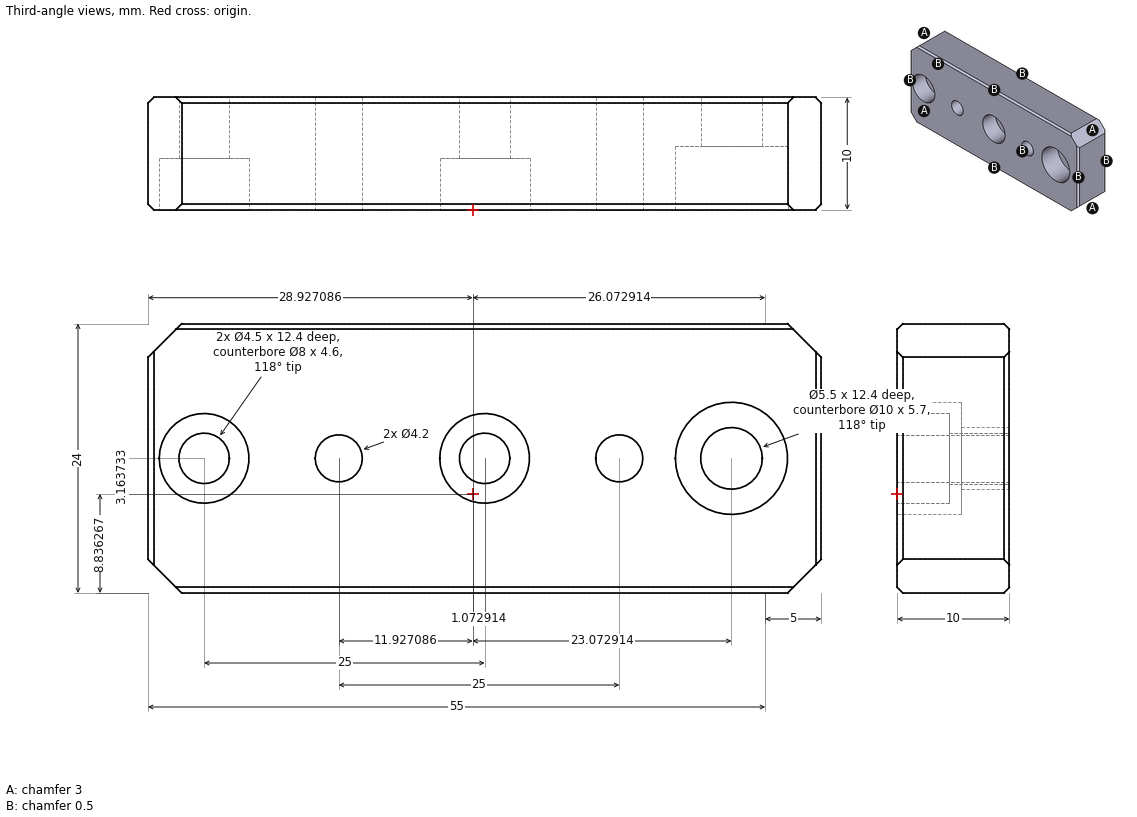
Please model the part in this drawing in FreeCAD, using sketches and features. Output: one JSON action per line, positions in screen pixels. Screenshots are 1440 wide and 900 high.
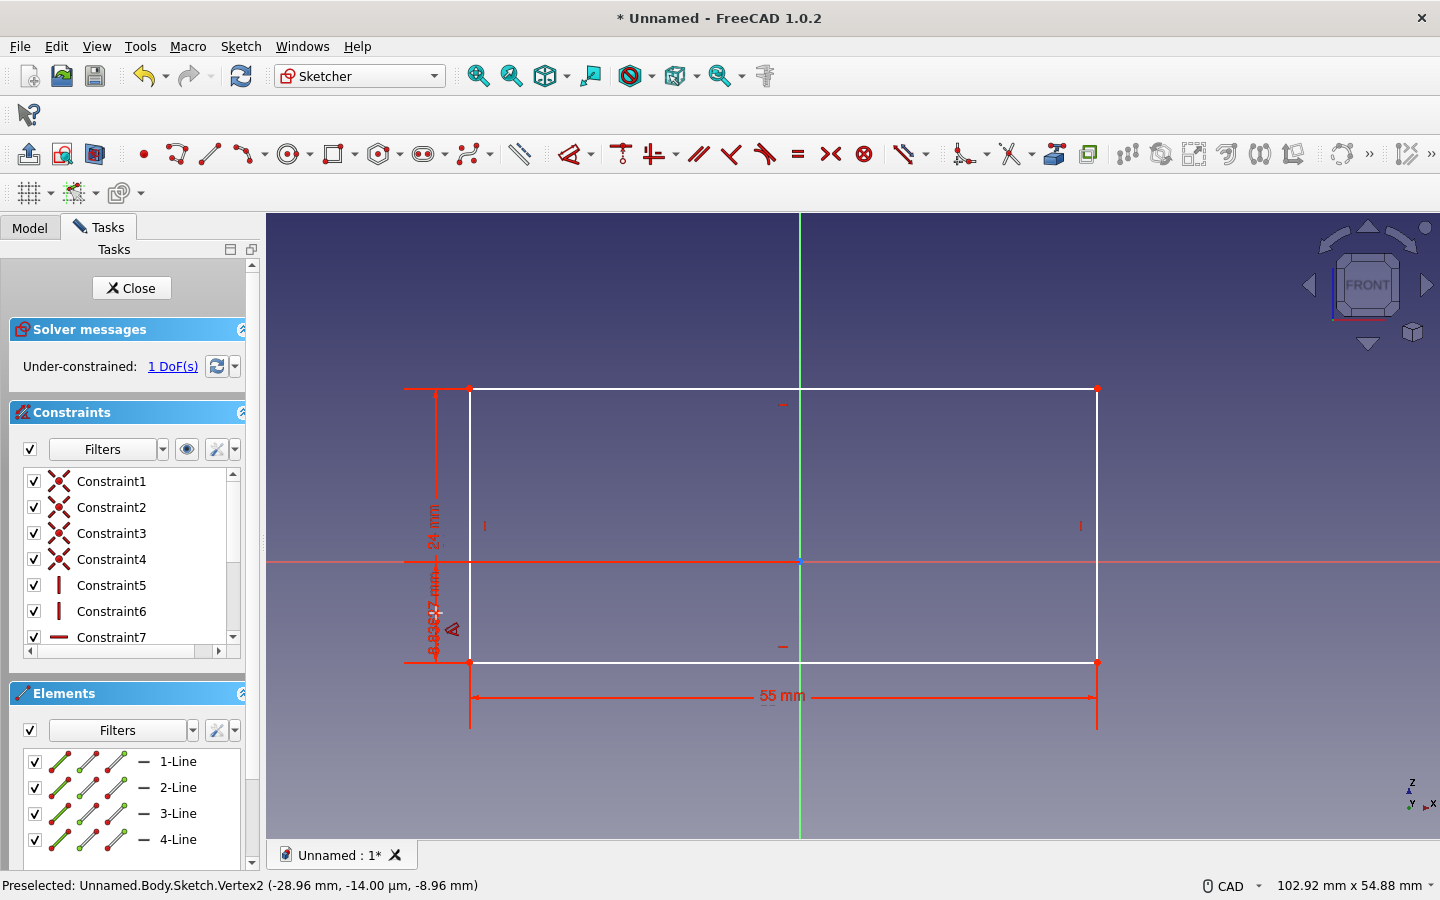
{"action": "left_click", "coordinate": [470, 389]}
{"action": "left_click", "coordinate": [635, 355]}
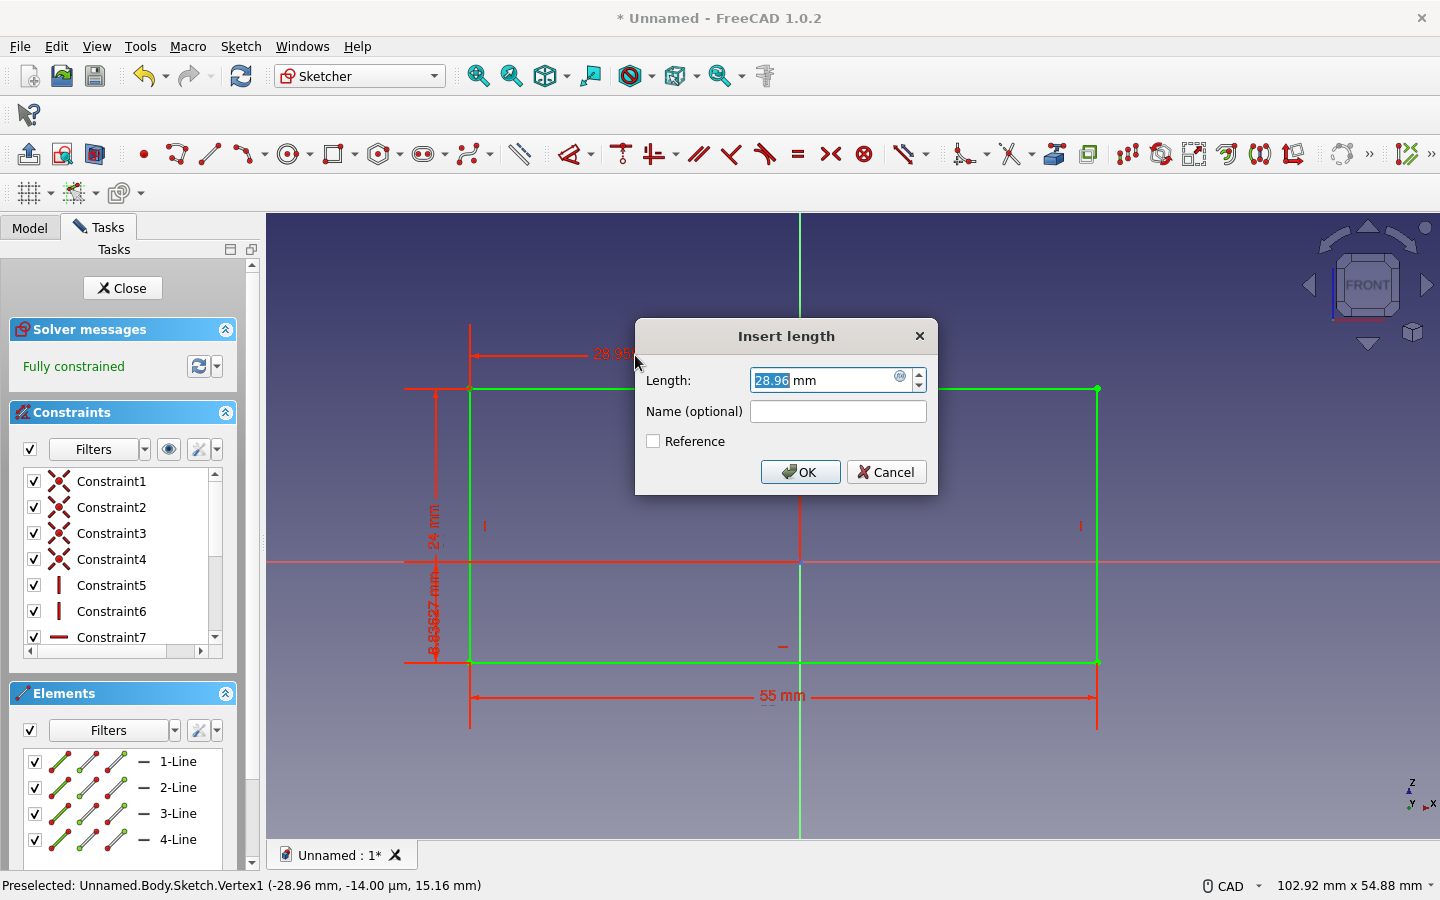
{"action": "type", "text": "28.927086"}
{"action": "key", "text": "Return"}
{"action": "key", "text": "Escape"}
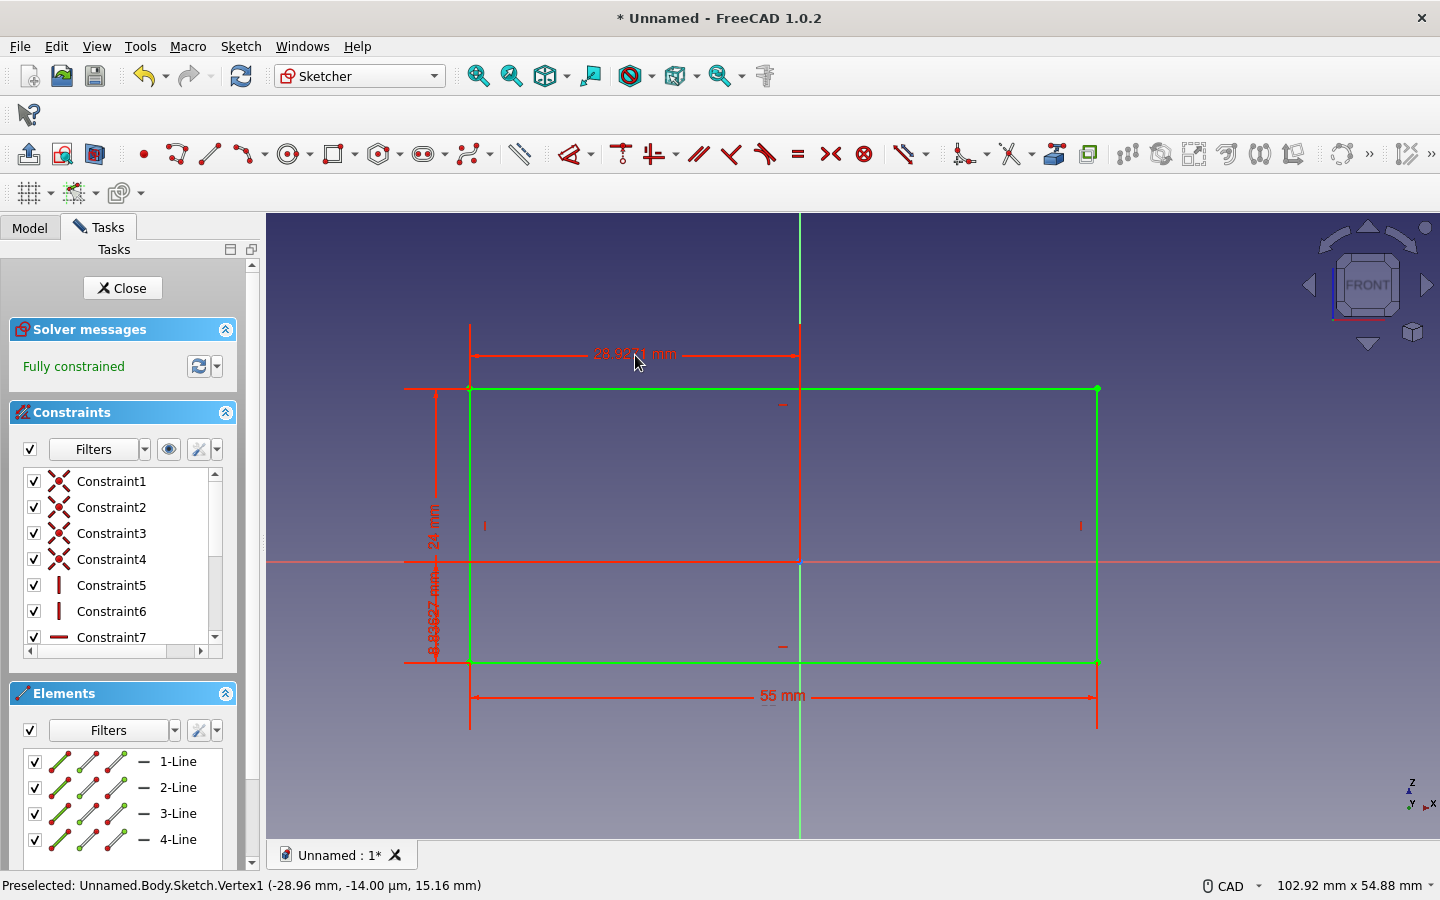
{"action": "left_click", "coordinate": [123, 288]}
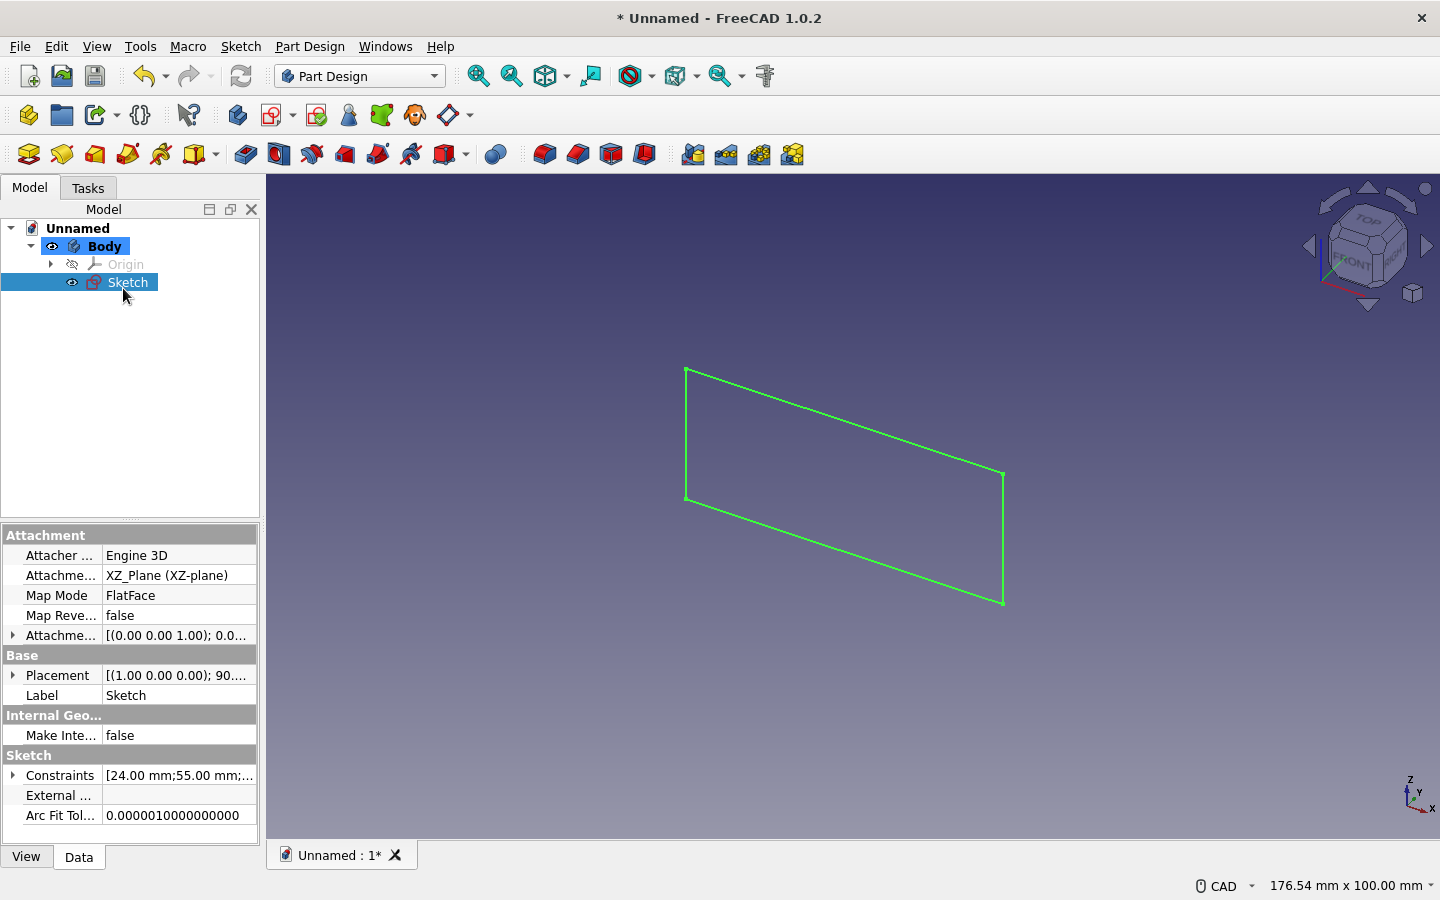
{"action": "left_click", "coordinate": [29, 154]}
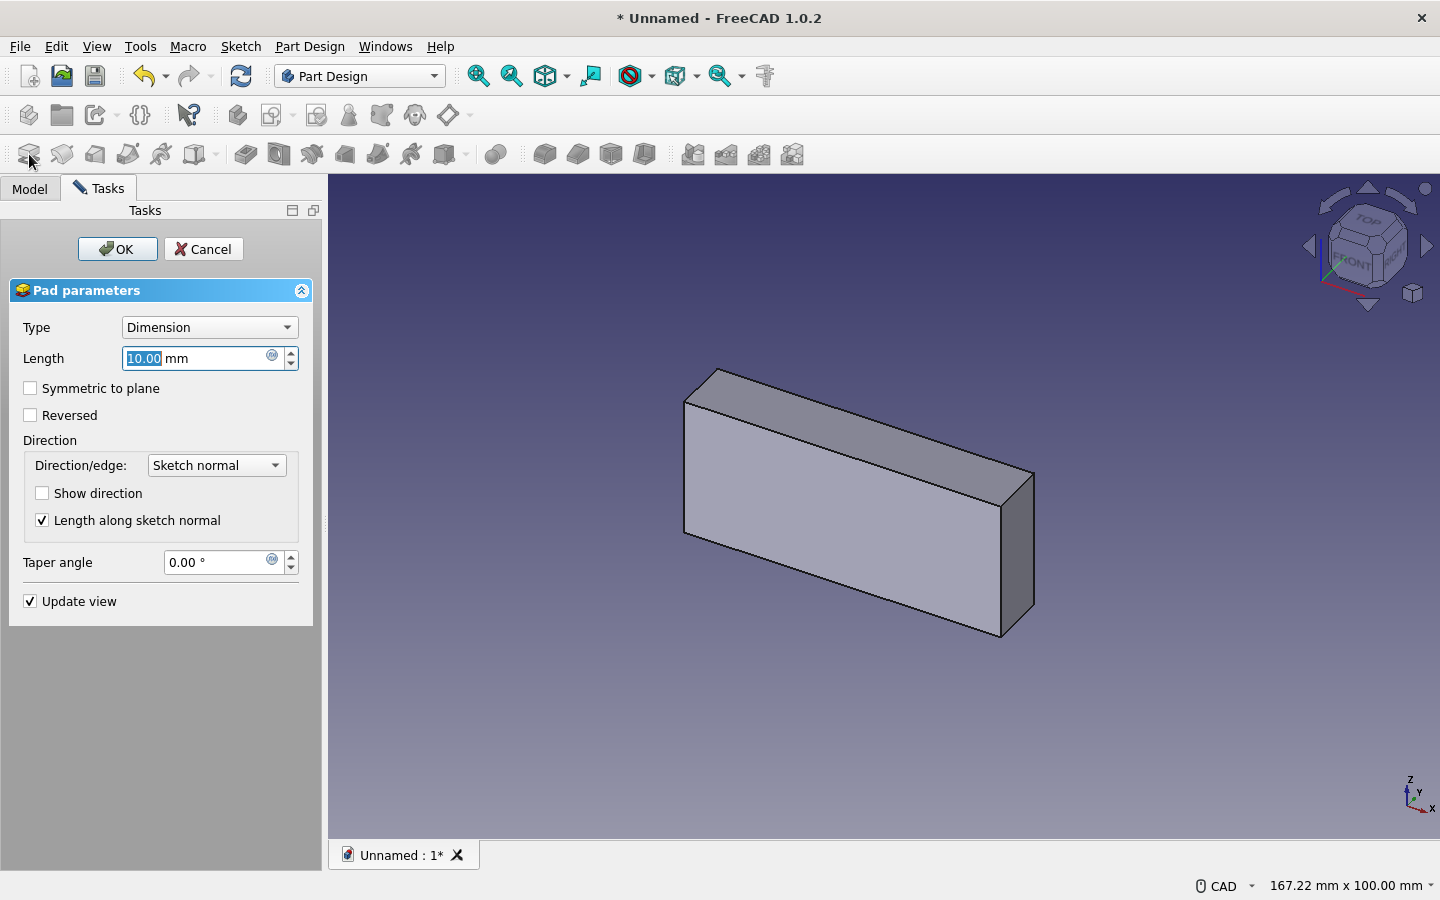
{"action": "type", "text": "10"}
{"action": "key", "text": "Tab"}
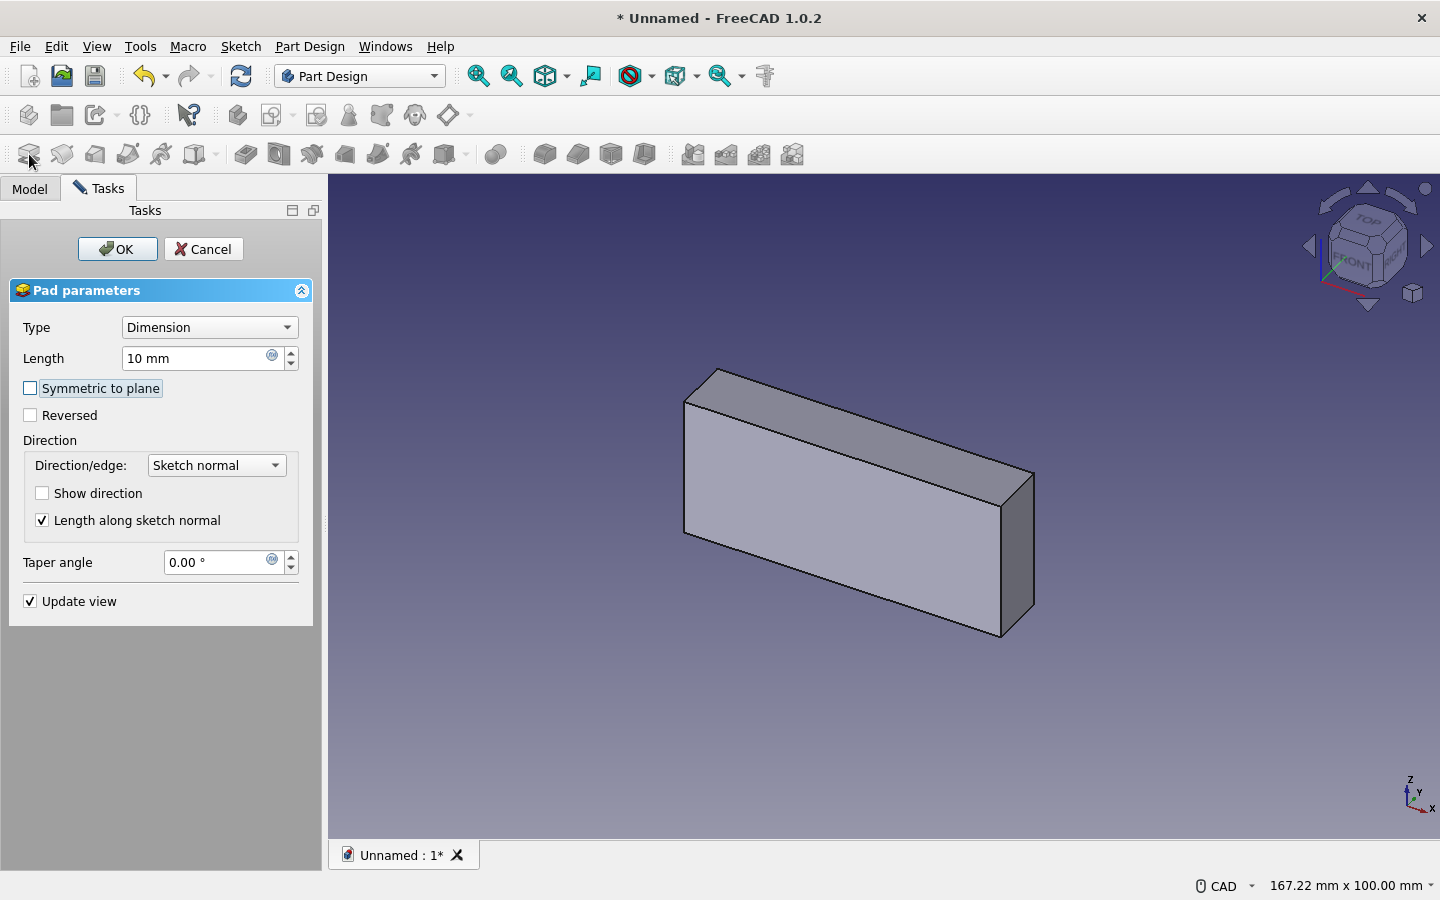
{"action": "left_click", "coordinate": [31, 415]}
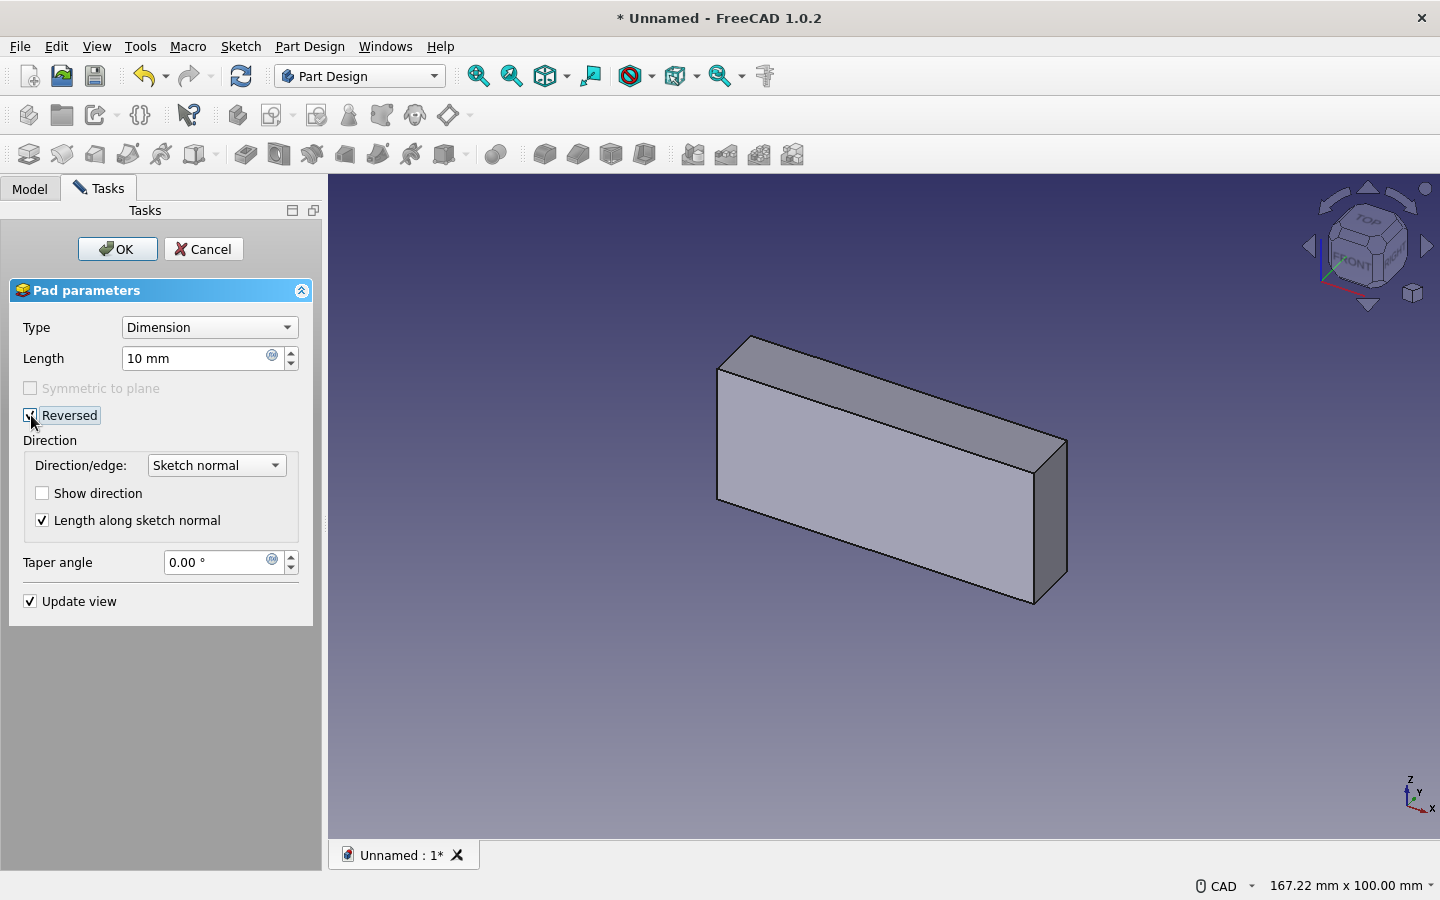
{"action": "left_click", "coordinate": [118, 249]}